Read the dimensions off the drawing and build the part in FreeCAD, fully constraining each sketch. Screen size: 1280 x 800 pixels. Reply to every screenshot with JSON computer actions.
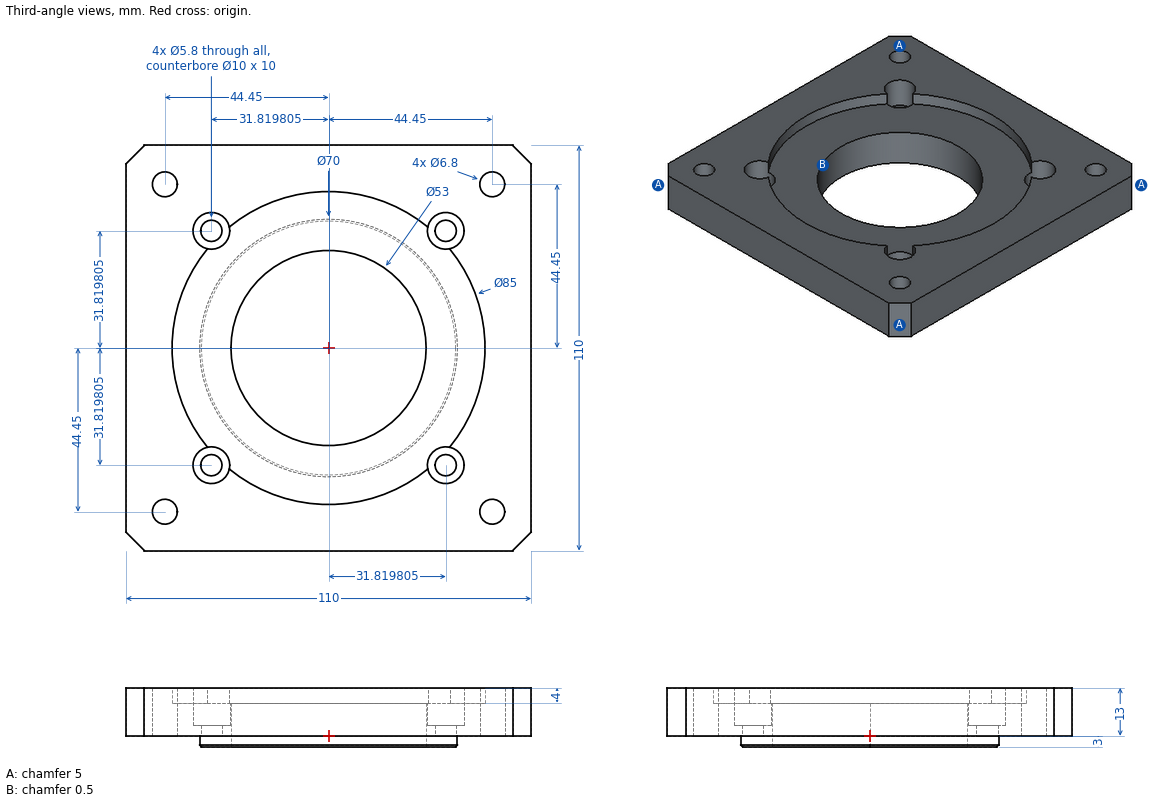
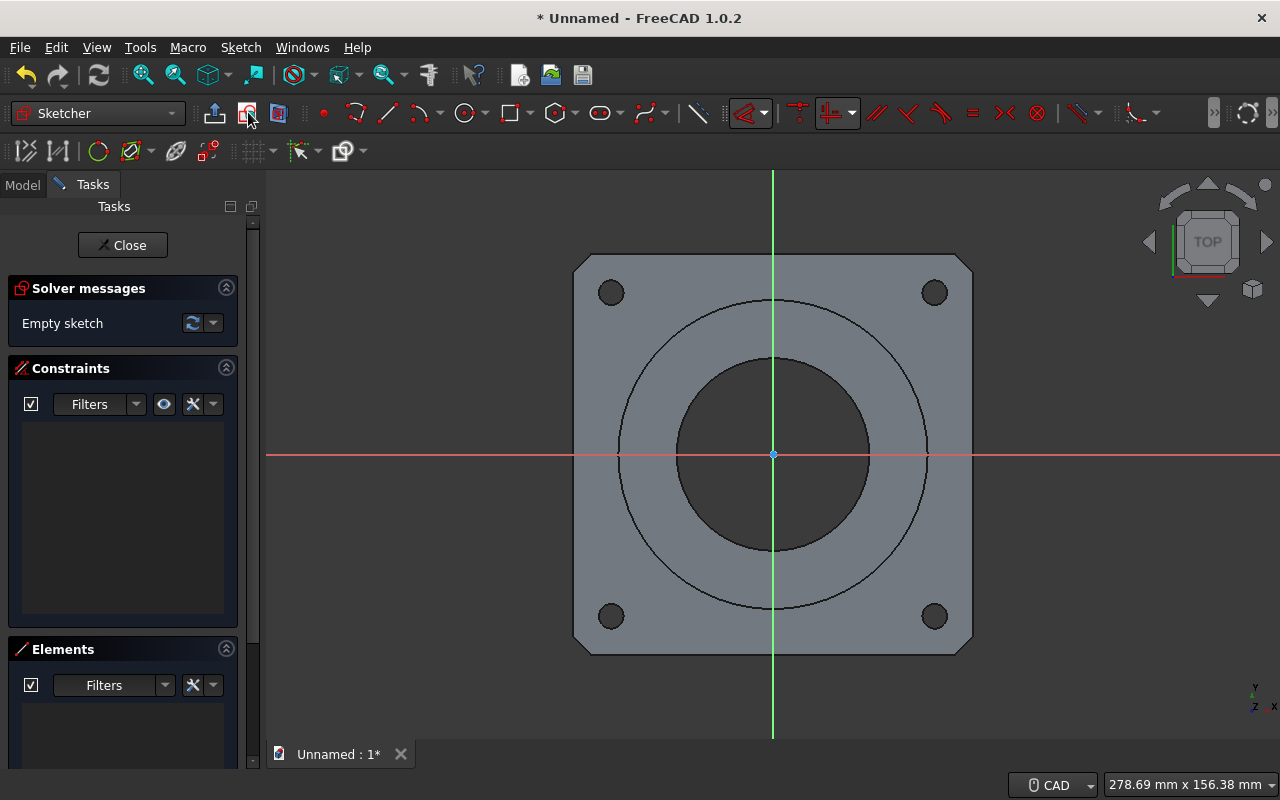
{"action": "scroll", "coordinate": [912, 455], "scroll_direction": "up", "scroll_amount": 2}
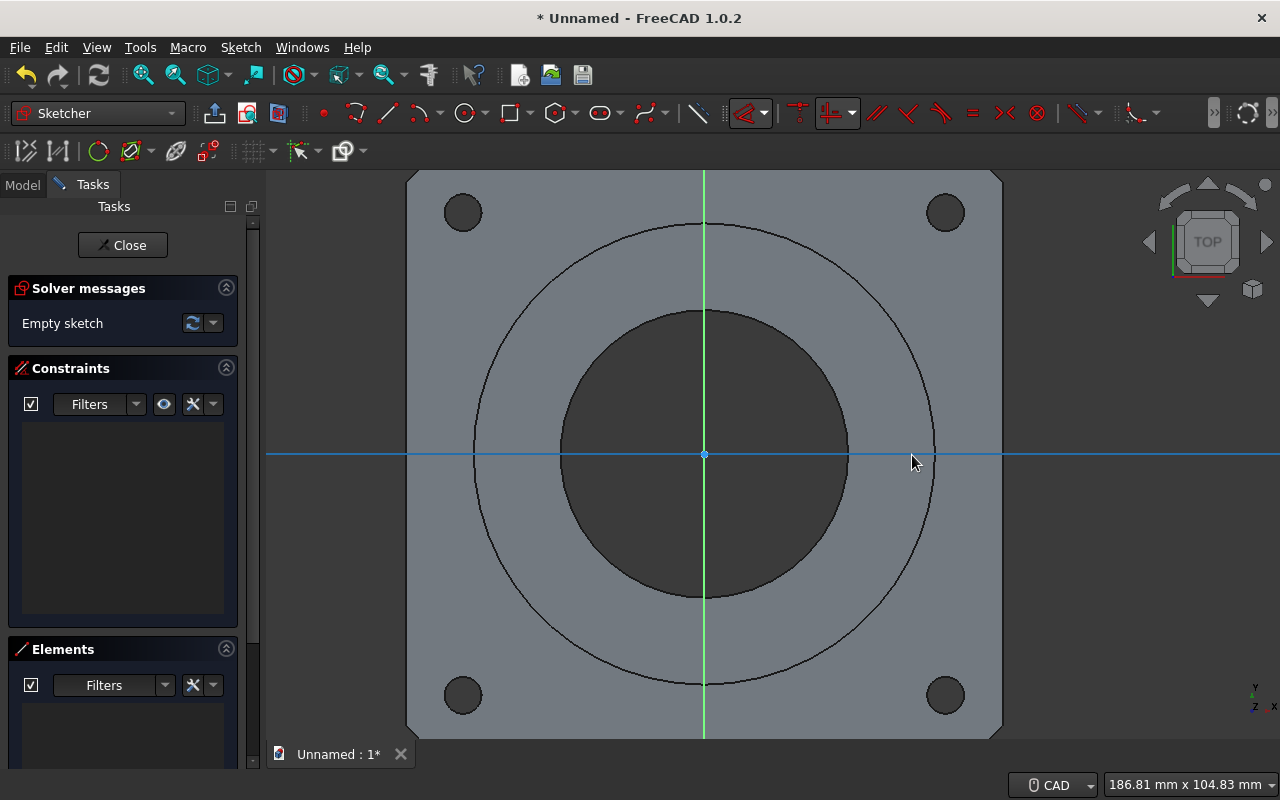
{"action": "key", "text": "g c"}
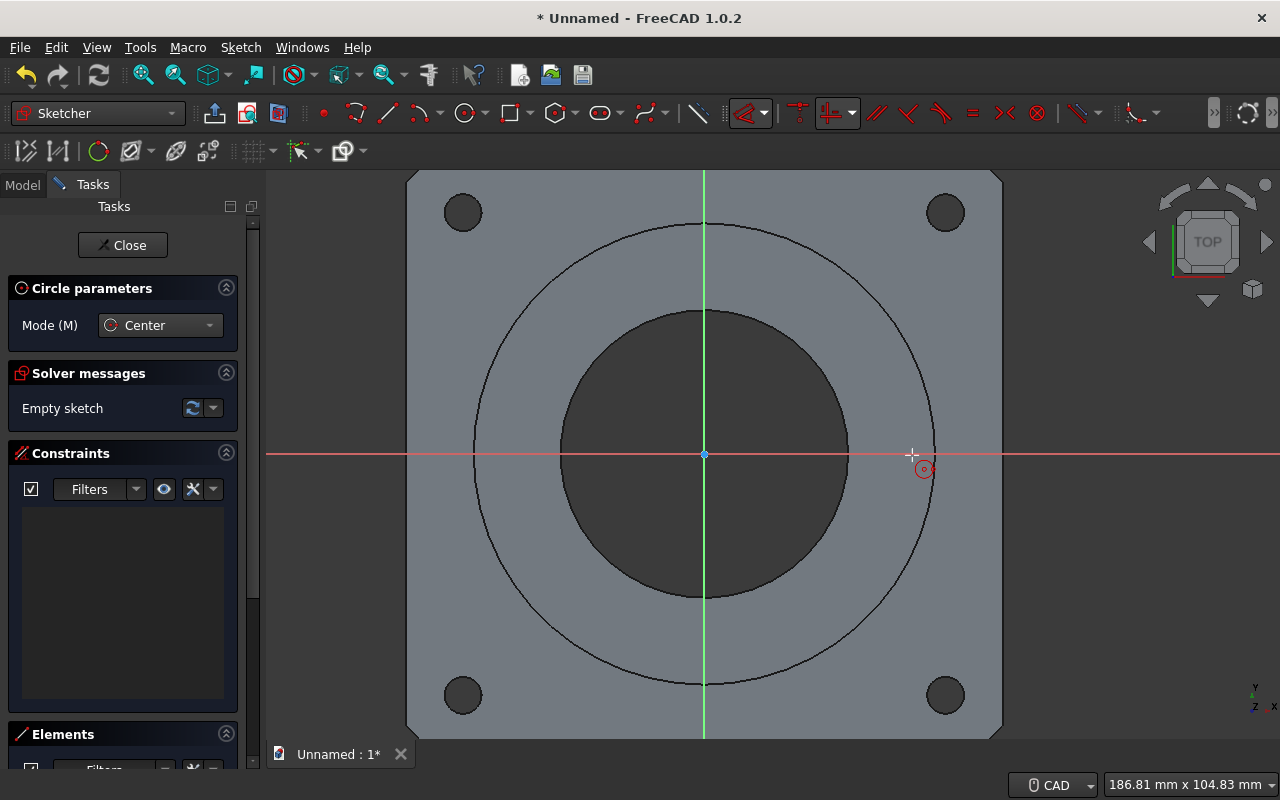
{"action": "scroll", "coordinate": [532, 281], "scroll_direction": "up", "scroll_amount": 2}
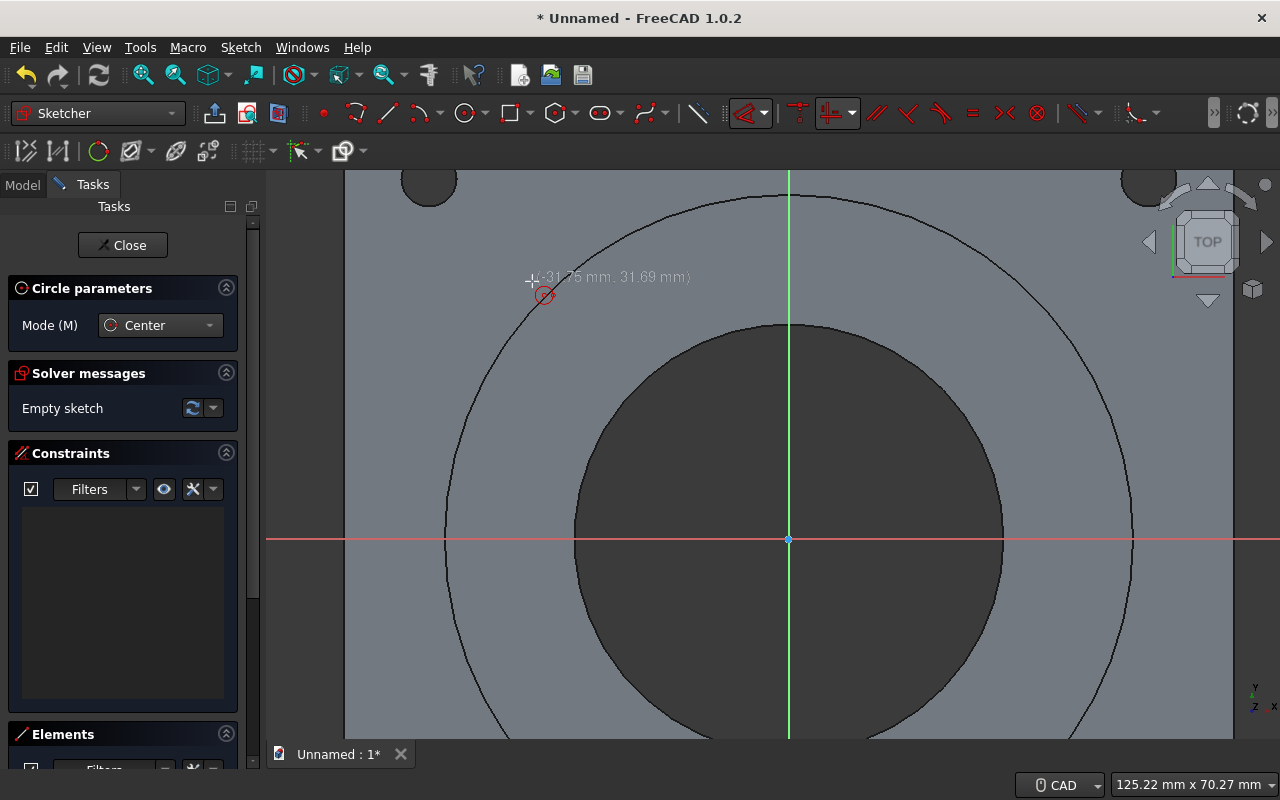
{"action": "left_click", "coordinate": [531, 281]}
{"action": "left_click", "coordinate": [548, 265]}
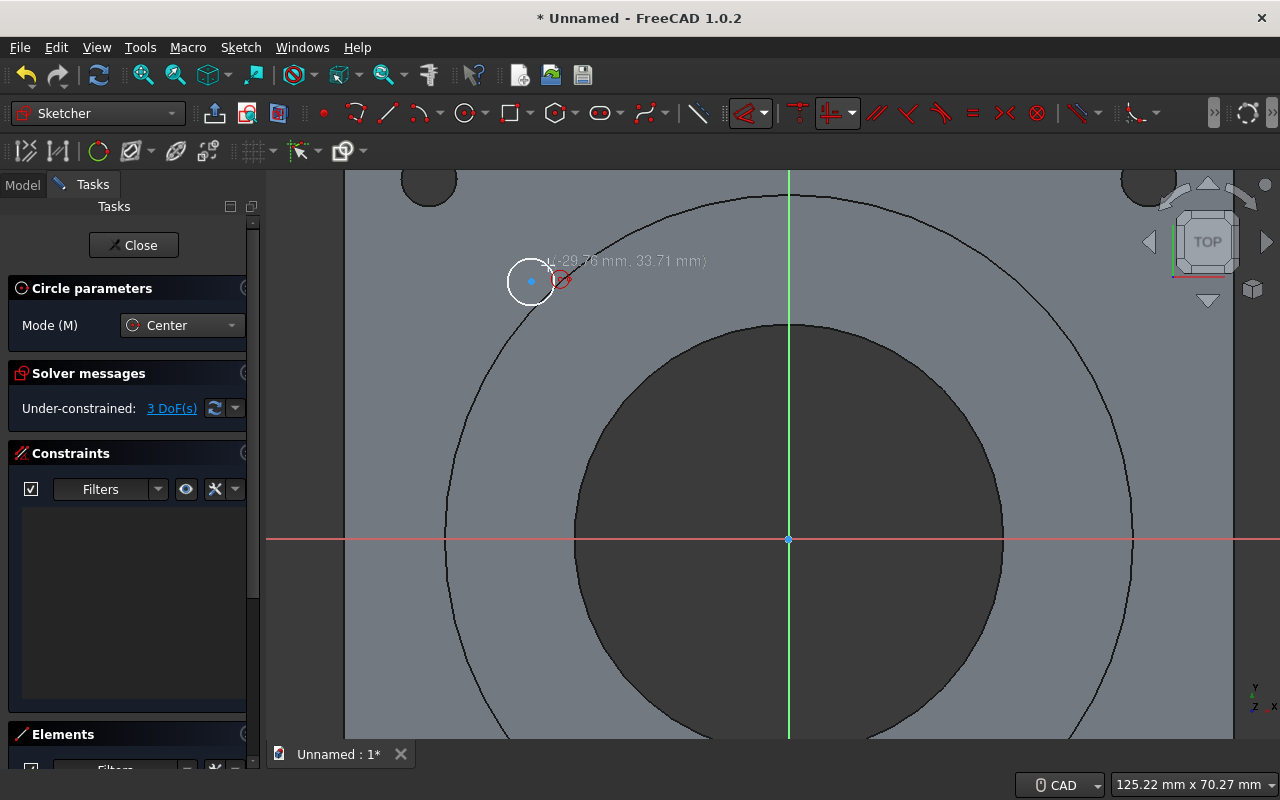
{"action": "scroll", "coordinate": [533, 283], "scroll_direction": "down", "scroll_amount": 2}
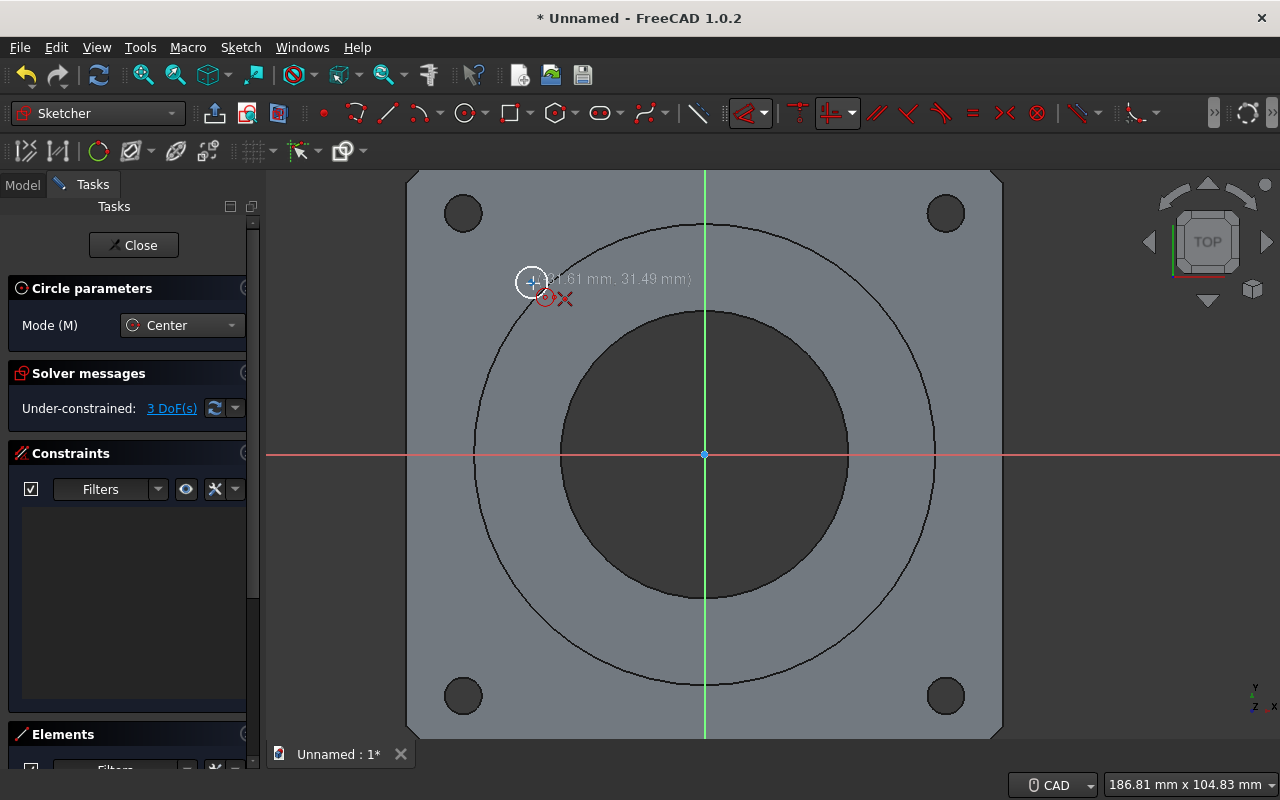
{"action": "scroll", "coordinate": [532, 627], "scroll_direction": "up", "scroll_amount": 2}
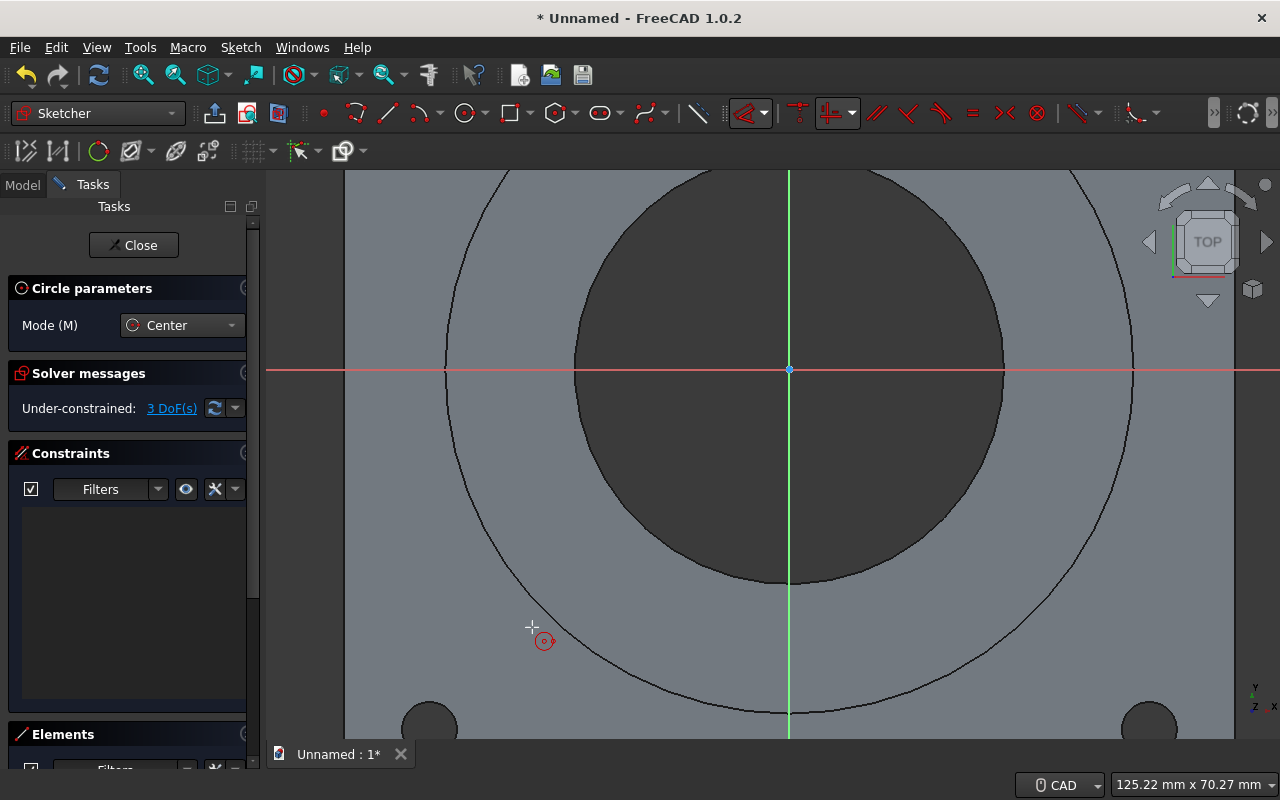
{"action": "left_click", "coordinate": [532, 627]}
{"action": "left_click", "coordinate": [548, 611]}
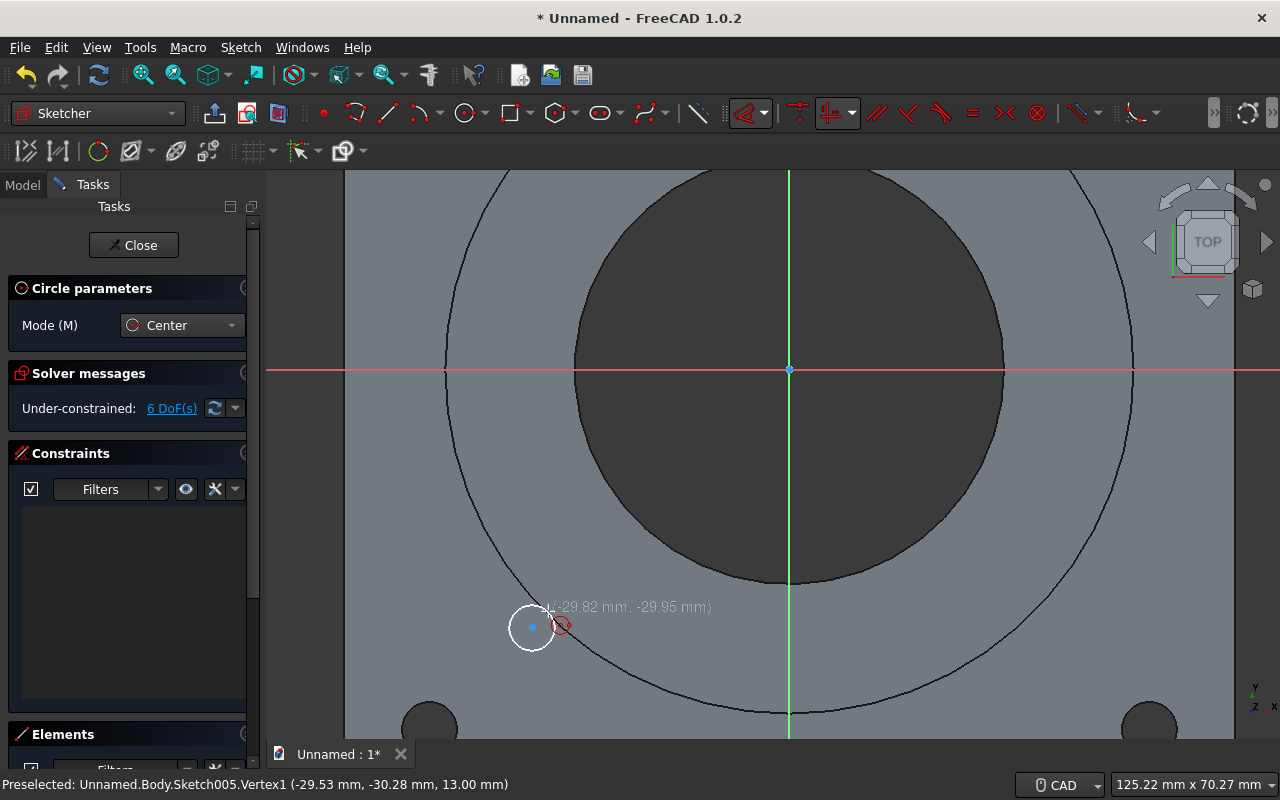
{"action": "left_click", "coordinate": [1047, 627]}
{"action": "left_click", "coordinate": [1064, 611]}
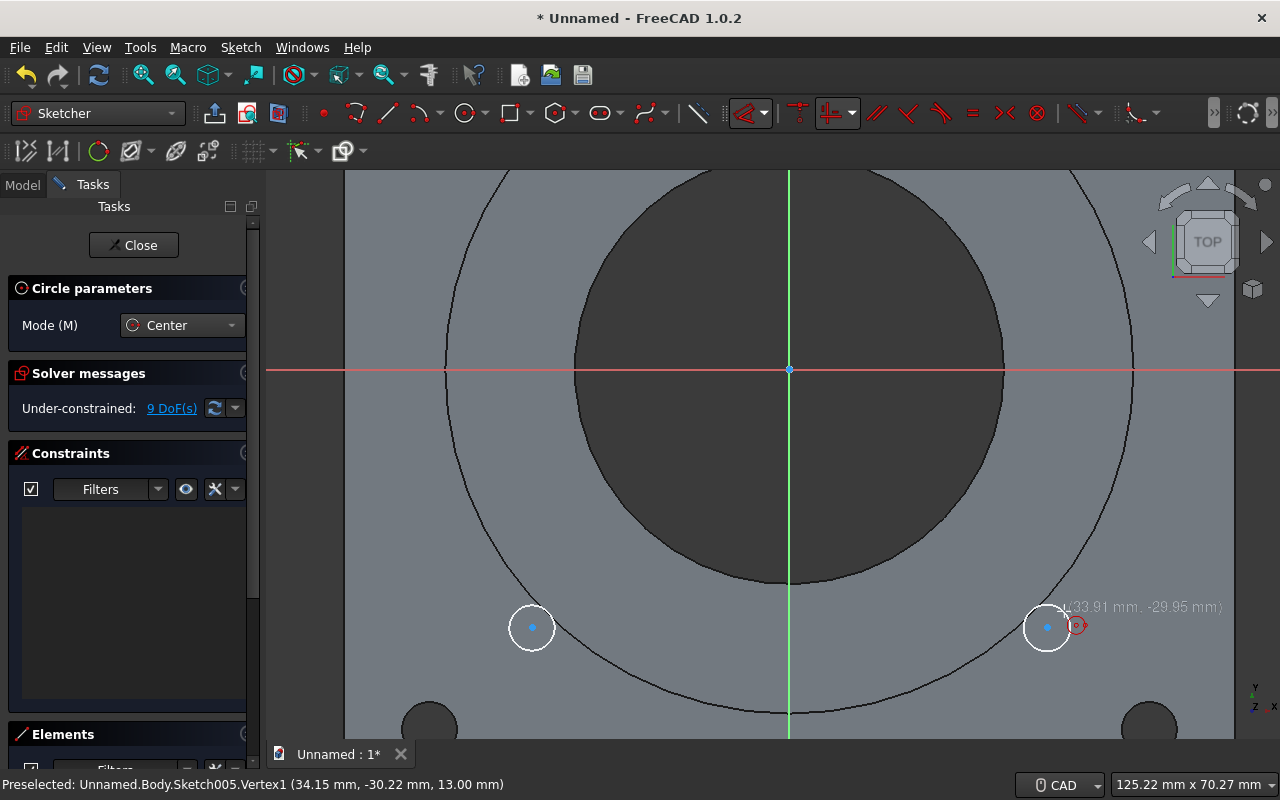
{"action": "scroll", "coordinate": [532, 627], "scroll_direction": "down", "scroll_amount": 2}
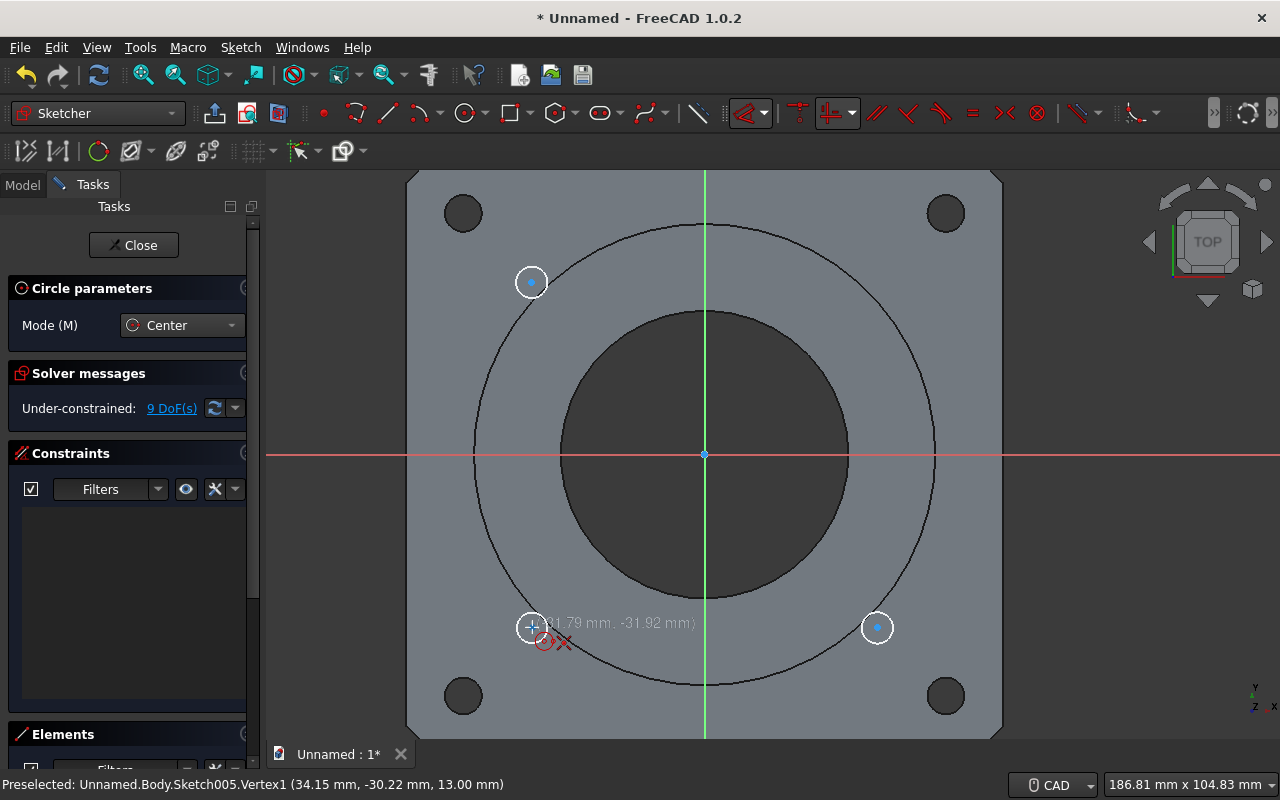
{"action": "scroll", "coordinate": [877, 282], "scroll_direction": "up", "scroll_amount": 2}